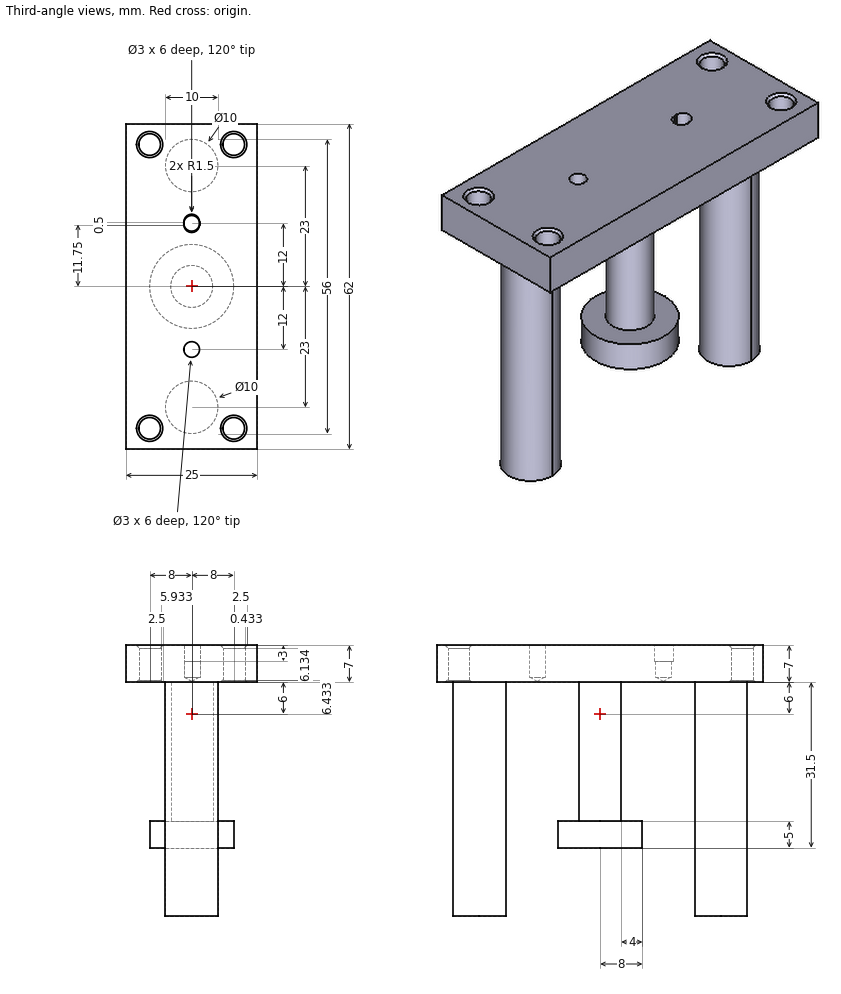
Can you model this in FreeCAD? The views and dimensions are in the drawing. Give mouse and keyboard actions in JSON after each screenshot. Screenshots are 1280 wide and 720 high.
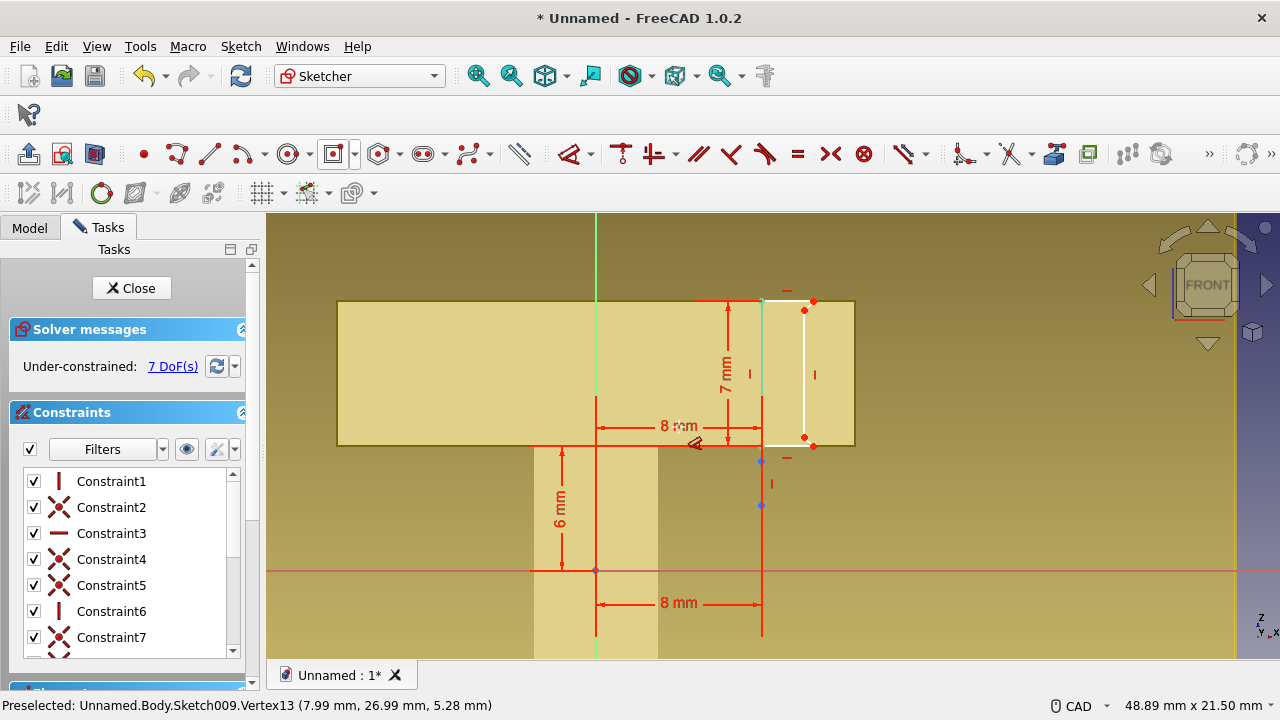
{"action": "left_click", "coordinate": [777, 301]}
{"action": "left_click", "coordinate": [788, 267]}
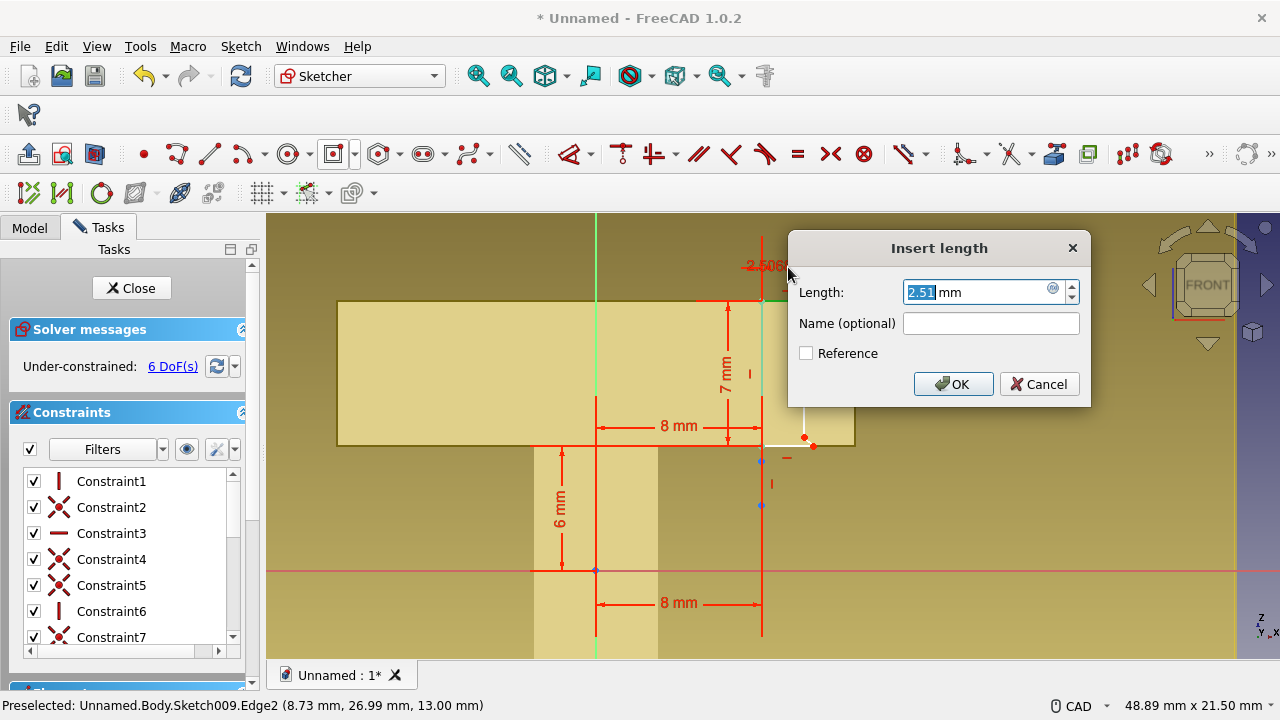
{"action": "type", "text": "2.5"}
{"action": "key", "text": "Return"}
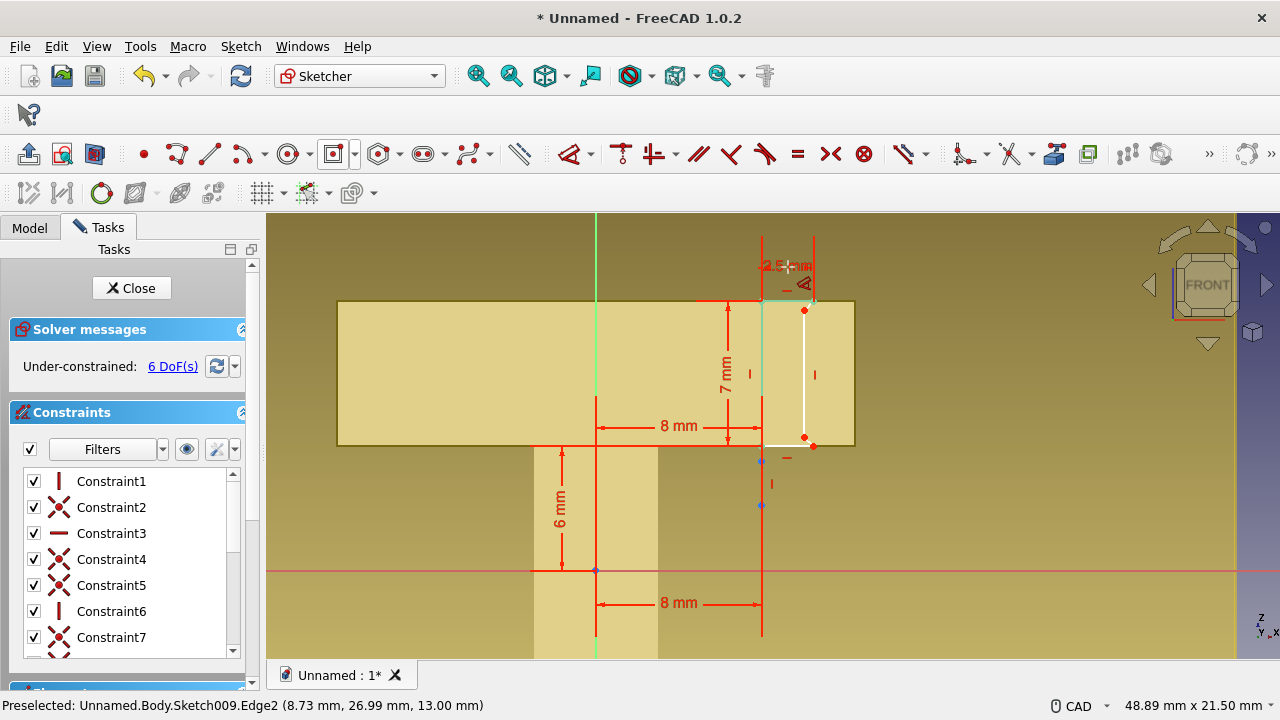
{"action": "scroll", "coordinate": [798, 446], "scroll_direction": "up", "scroll_amount": 2}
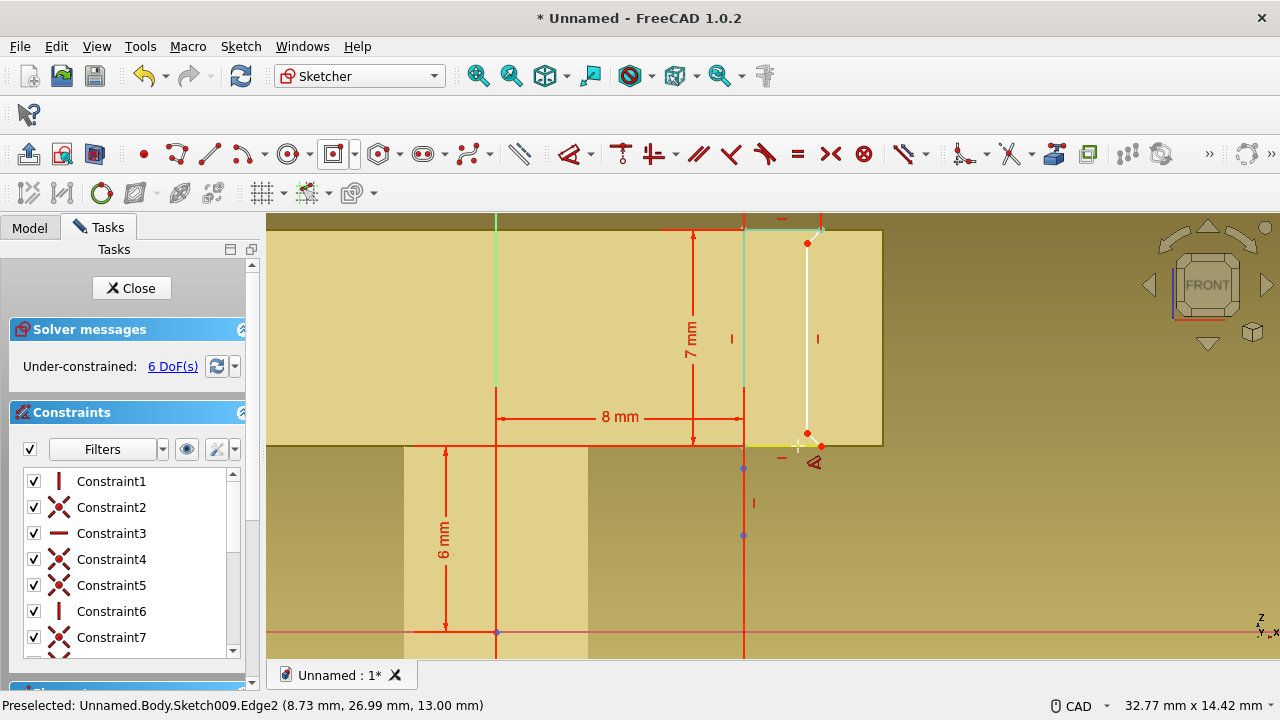
{"action": "left_click", "coordinate": [798, 446]}
{"action": "left_click", "coordinate": [783, 480]}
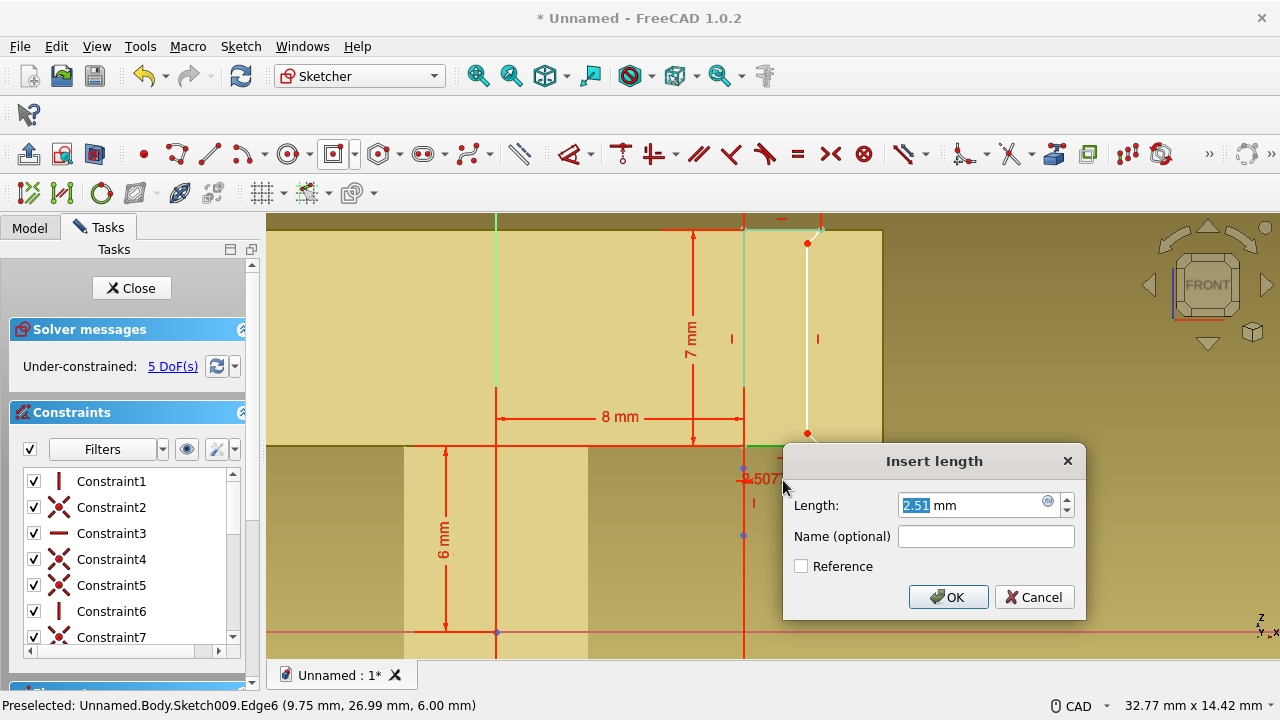
{"action": "type", "text": "2.5"}
{"action": "key", "text": "Return"}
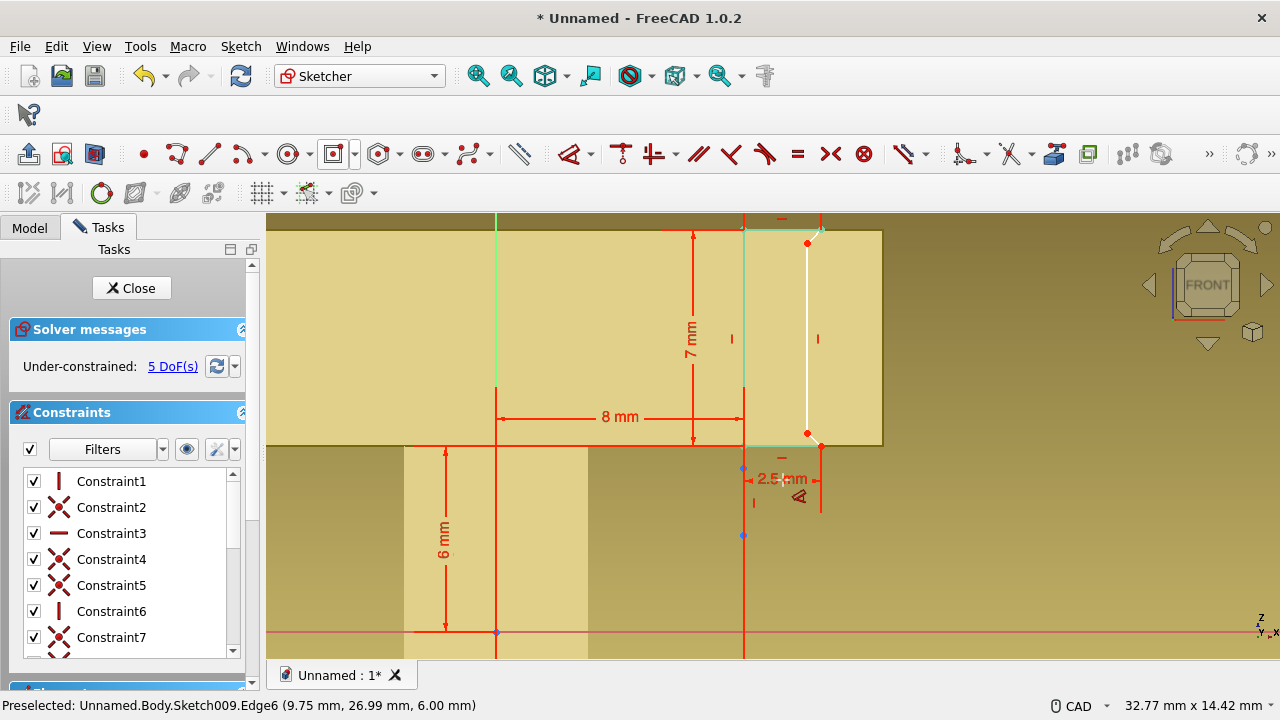
{"action": "left_click", "coordinate": [807, 301]}
{"action": "left_click", "coordinate": [841, 339]}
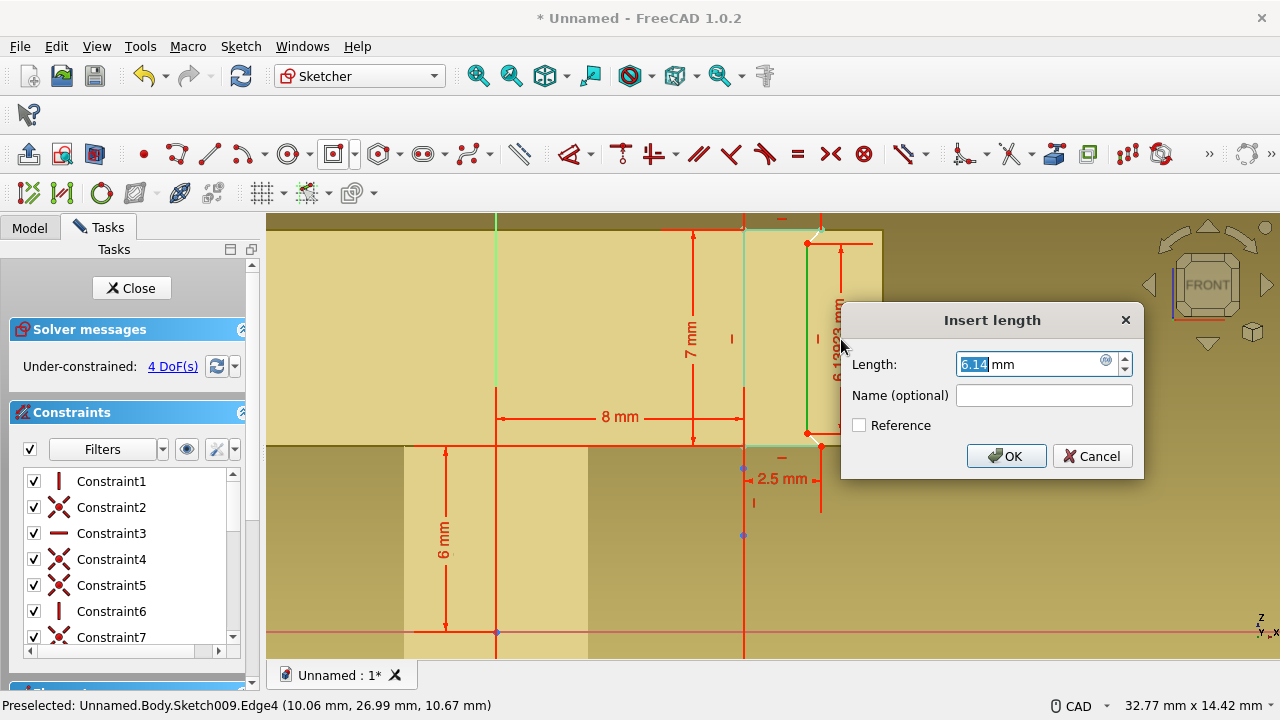
{"action": "type", "text": "6.134"}
{"action": "key", "text": "Return"}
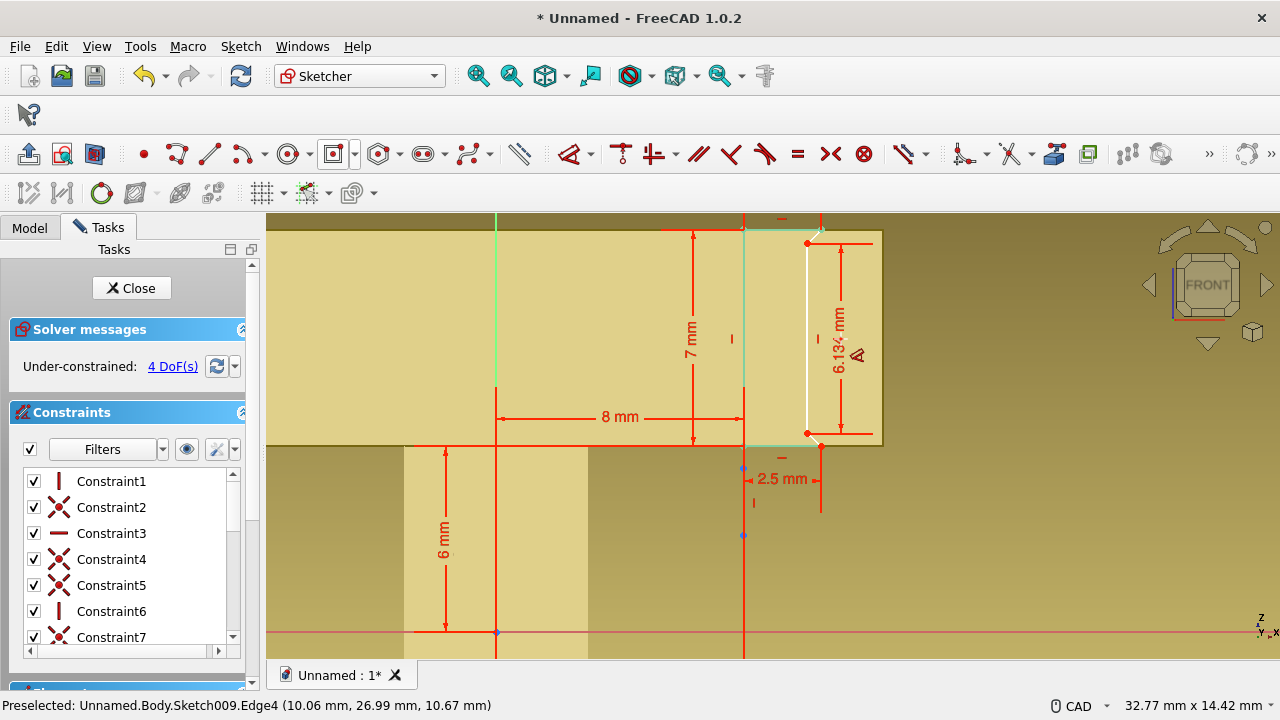
{"action": "left_click", "coordinate": [807, 434]}
{"action": "left_click", "coordinate": [462, 487]}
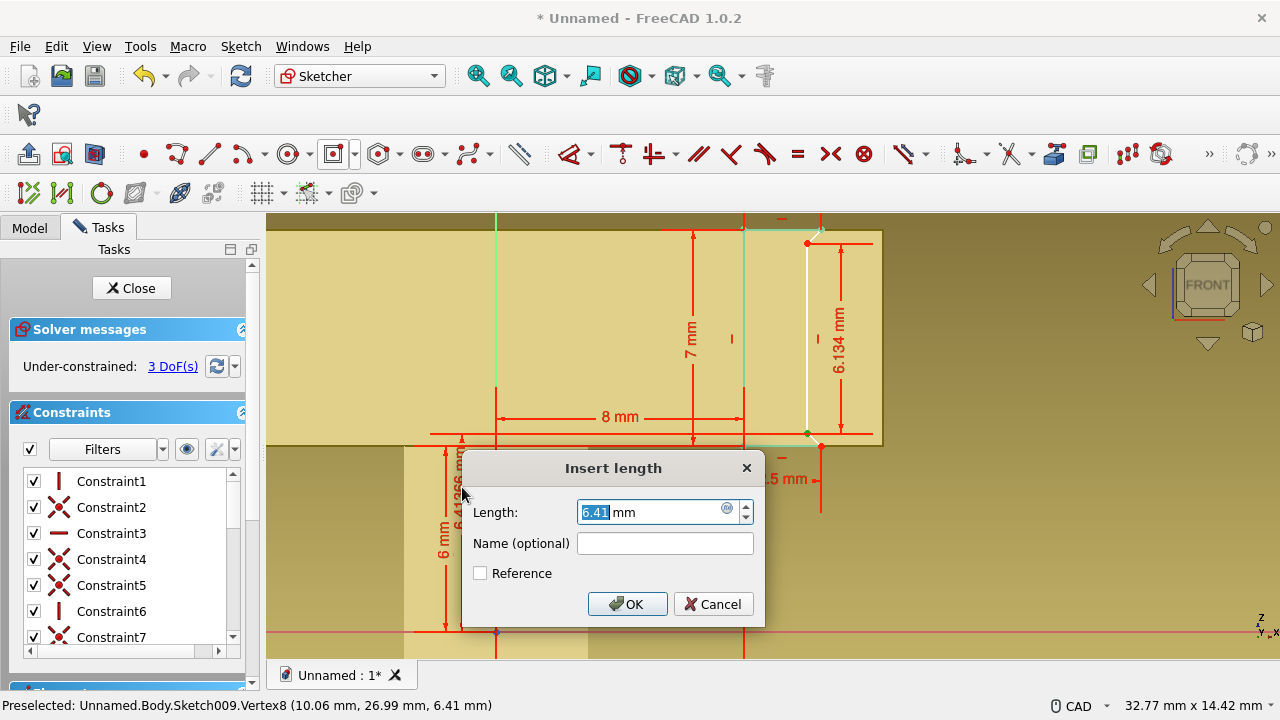
{"action": "type", "text": "6.433"}
{"action": "key", "text": "Return"}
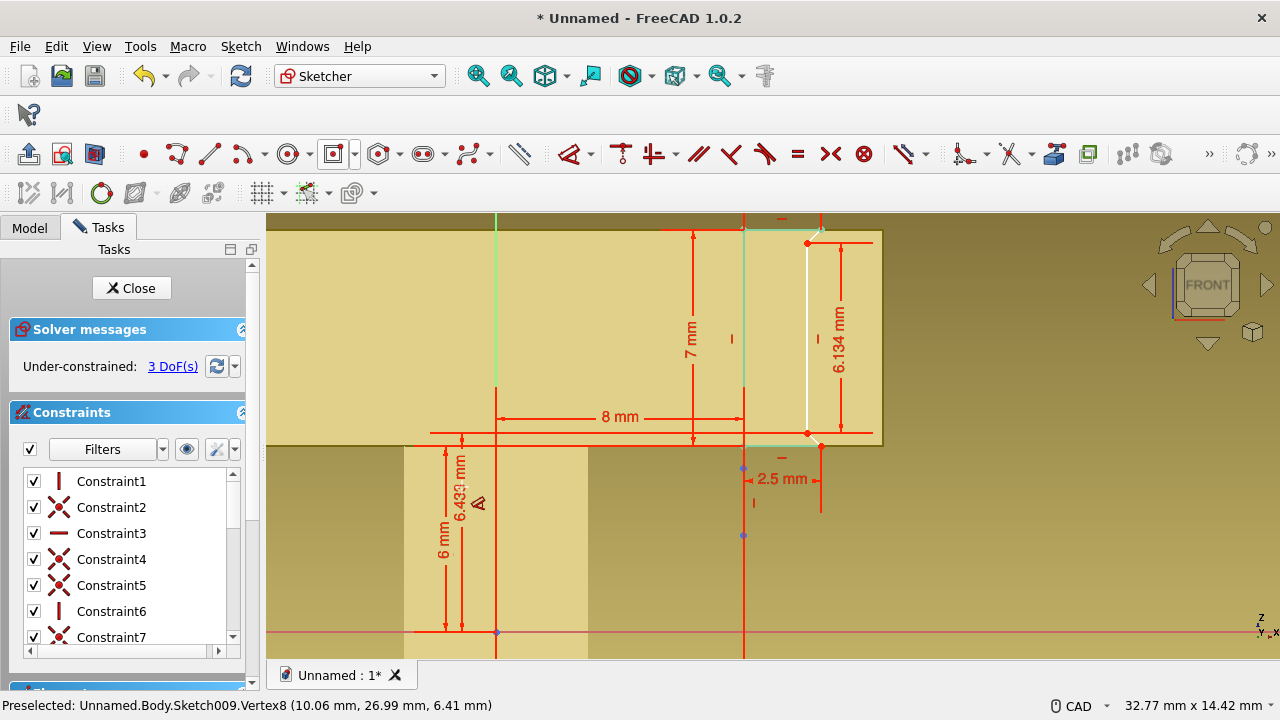
{"action": "scroll", "coordinate": [798, 446], "scroll_direction": "down", "scroll_amount": 2}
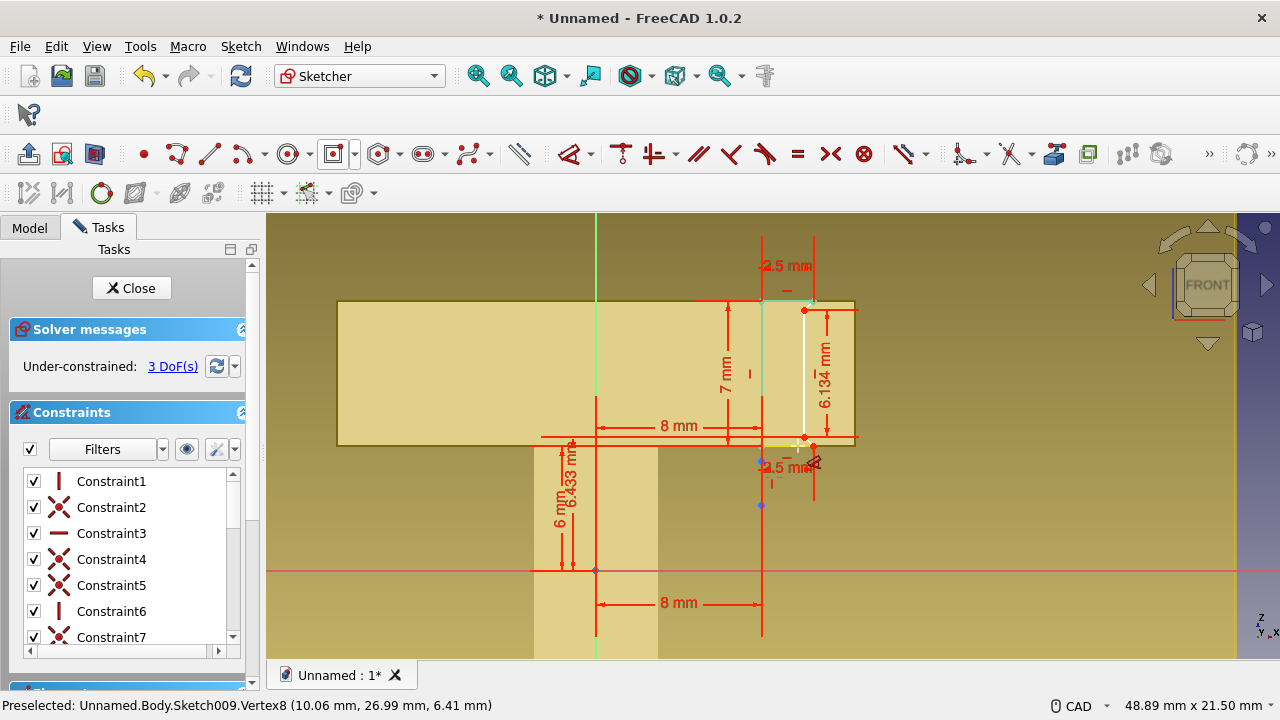
{"action": "scroll", "coordinate": [808, 307], "scroll_direction": "up", "scroll_amount": 8}